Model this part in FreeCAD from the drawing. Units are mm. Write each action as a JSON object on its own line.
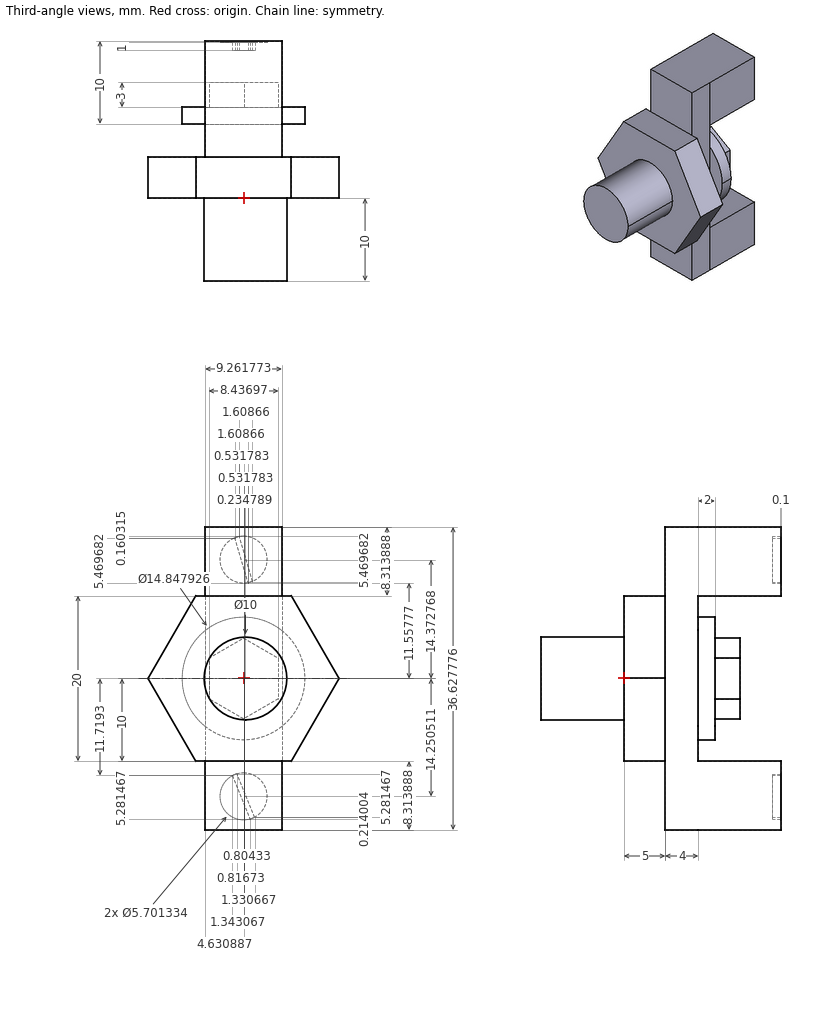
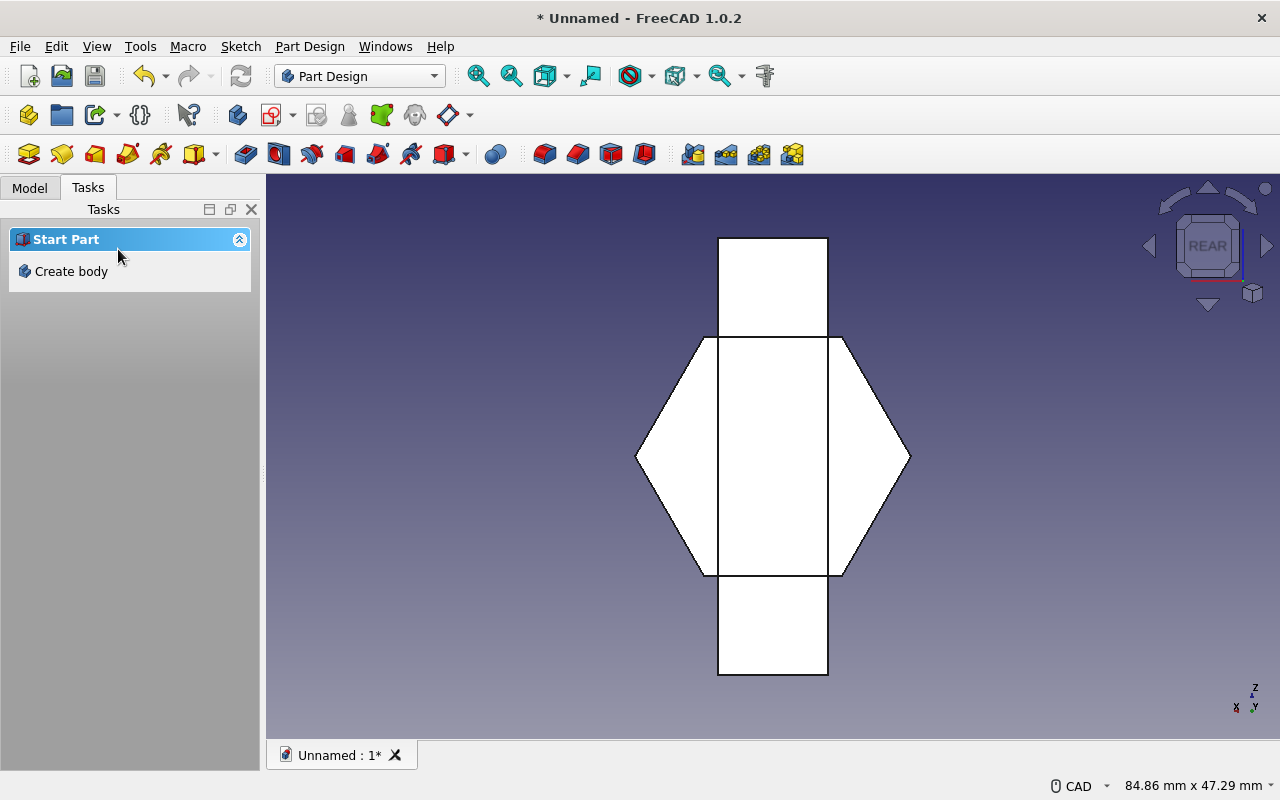
{"action": "left_click", "coordinate": [773, 455]}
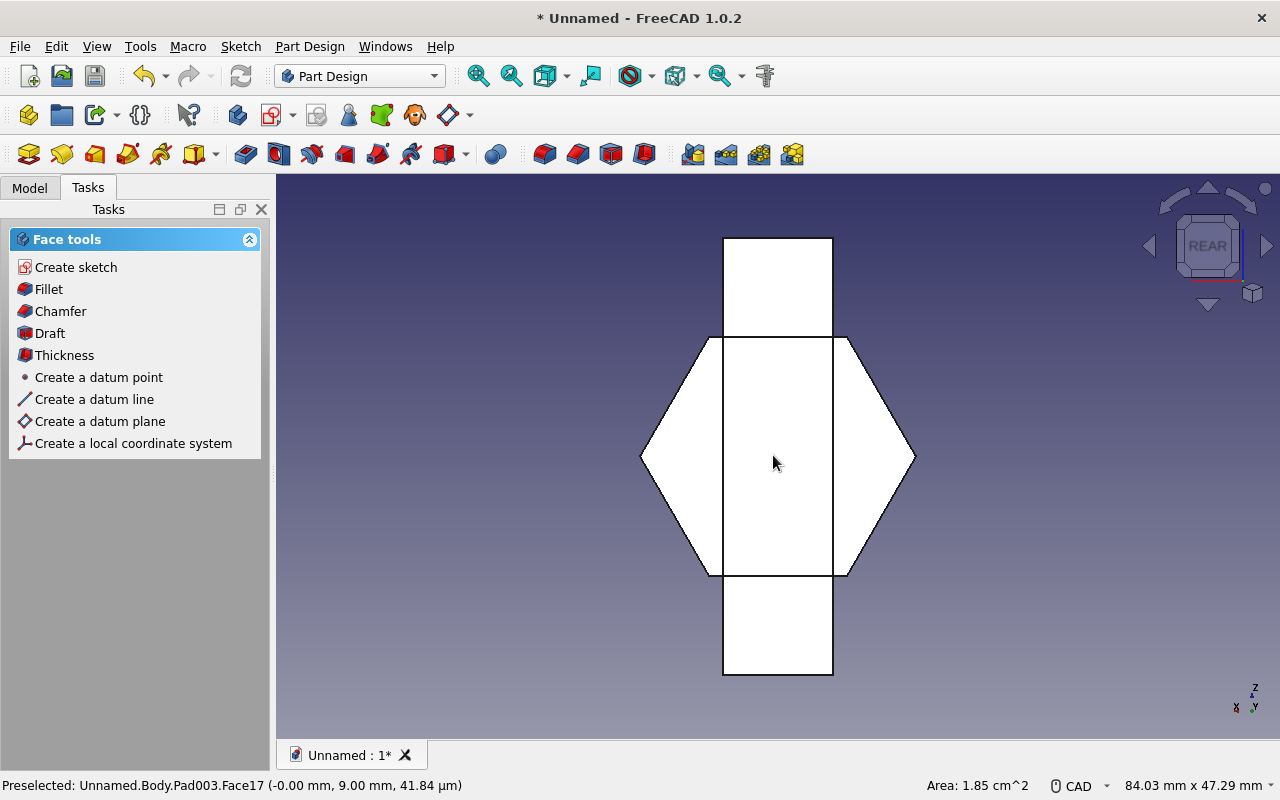
{"action": "left_click", "coordinate": [270, 116]}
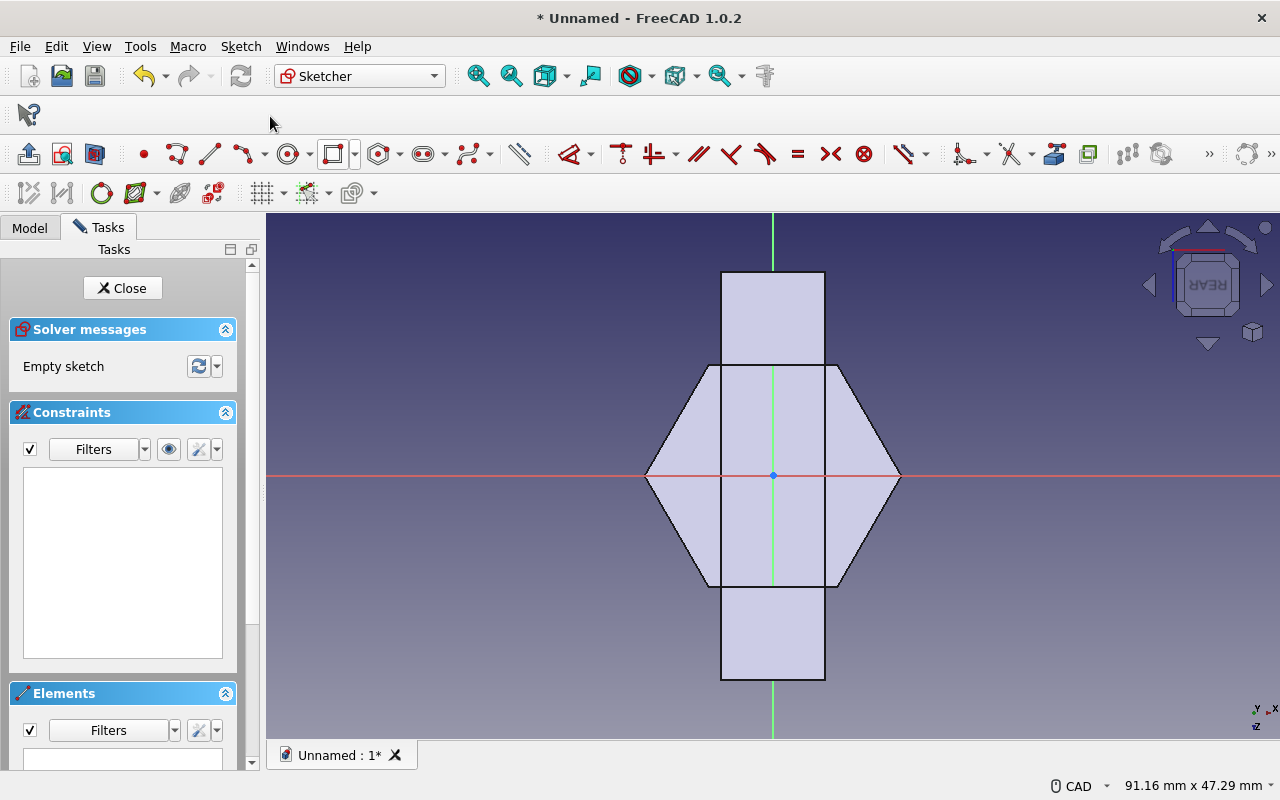
{"action": "scroll", "coordinate": [856, 476], "scroll_direction": "up", "scroll_amount": 3}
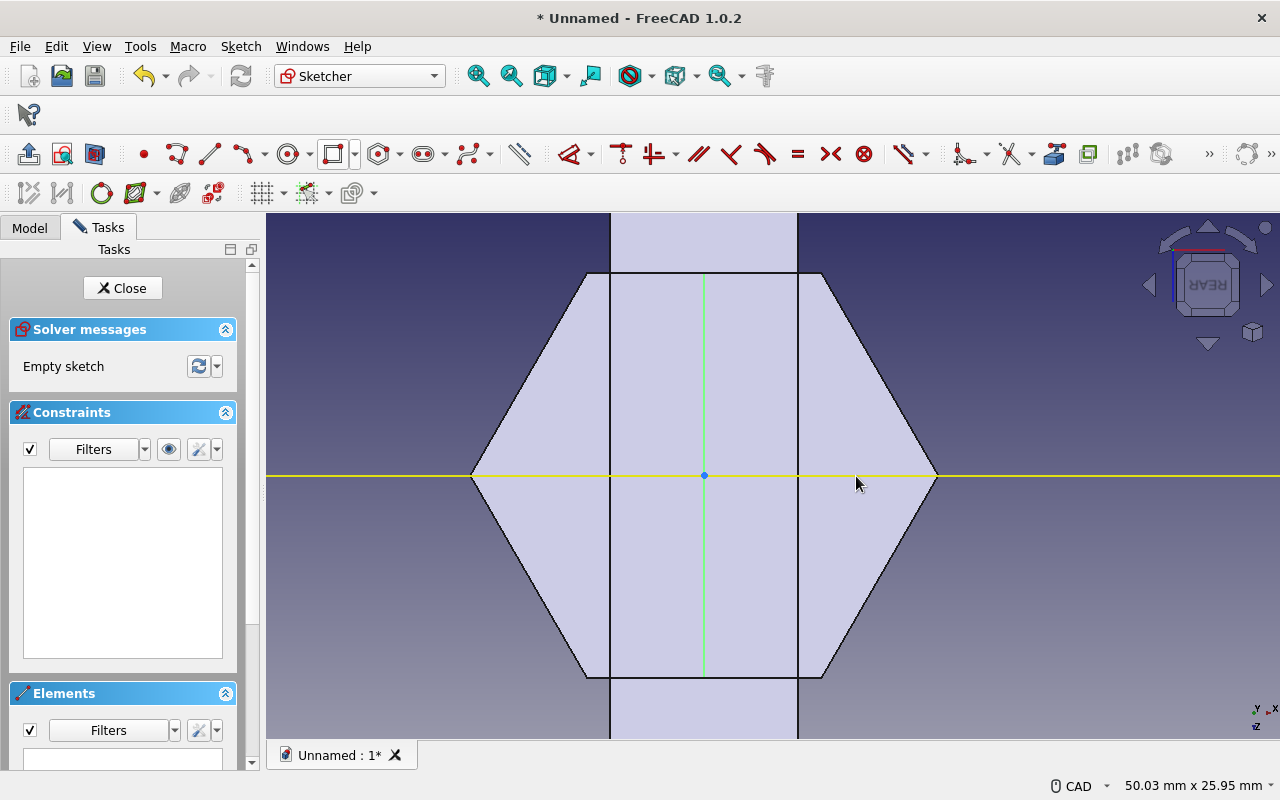
{"action": "left_click", "coordinate": [288, 154]}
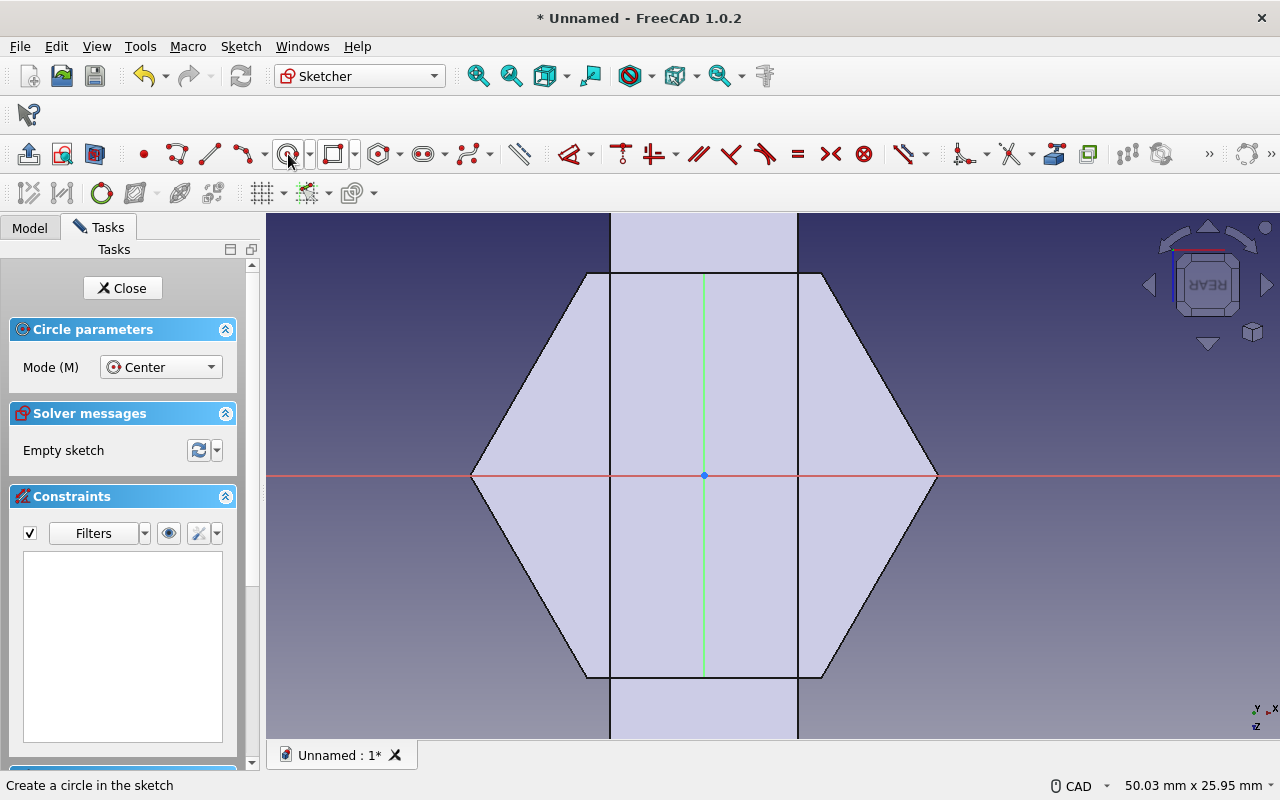
{"action": "left_click", "coordinate": [704, 476]}
{"action": "mouse_move", "coordinate": [811, 369]}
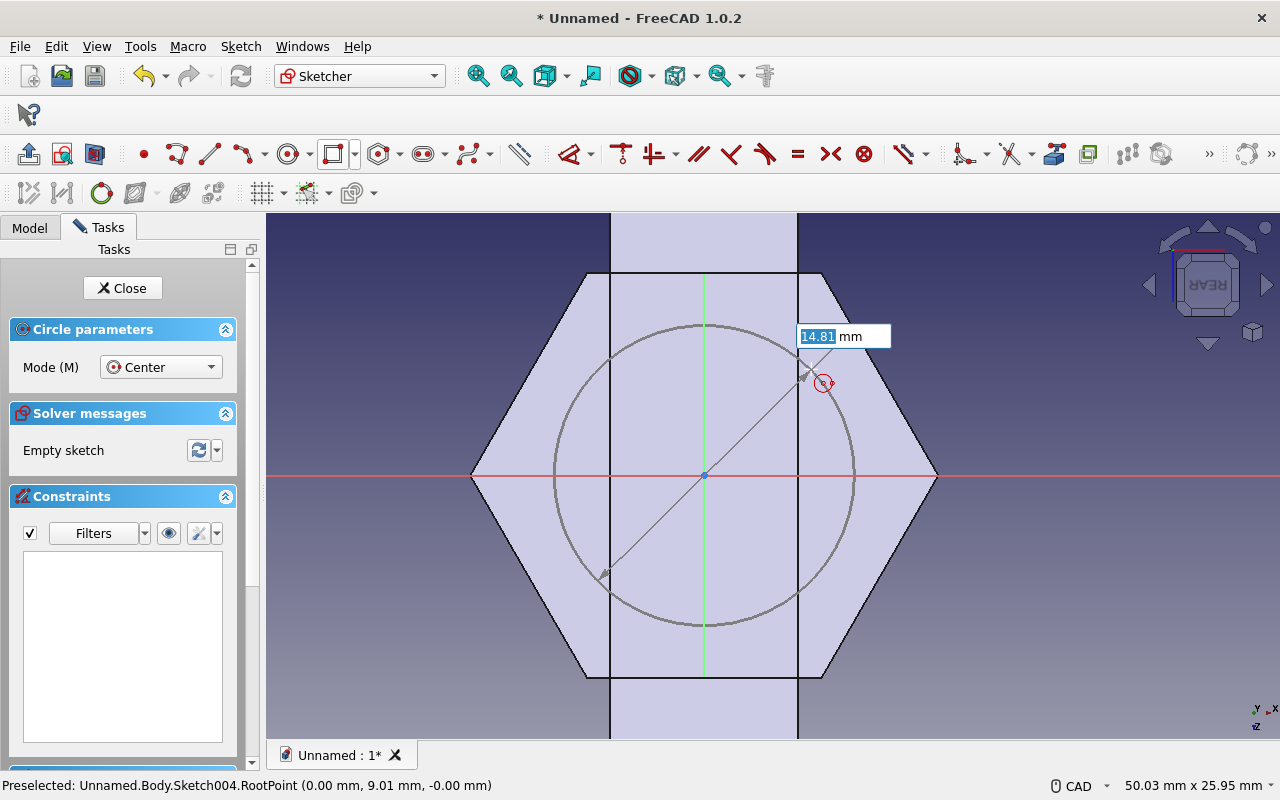
{"action": "type", "text": "14.847926"}
{"action": "key", "text": "Return"}
{"action": "key", "text": "Escape"}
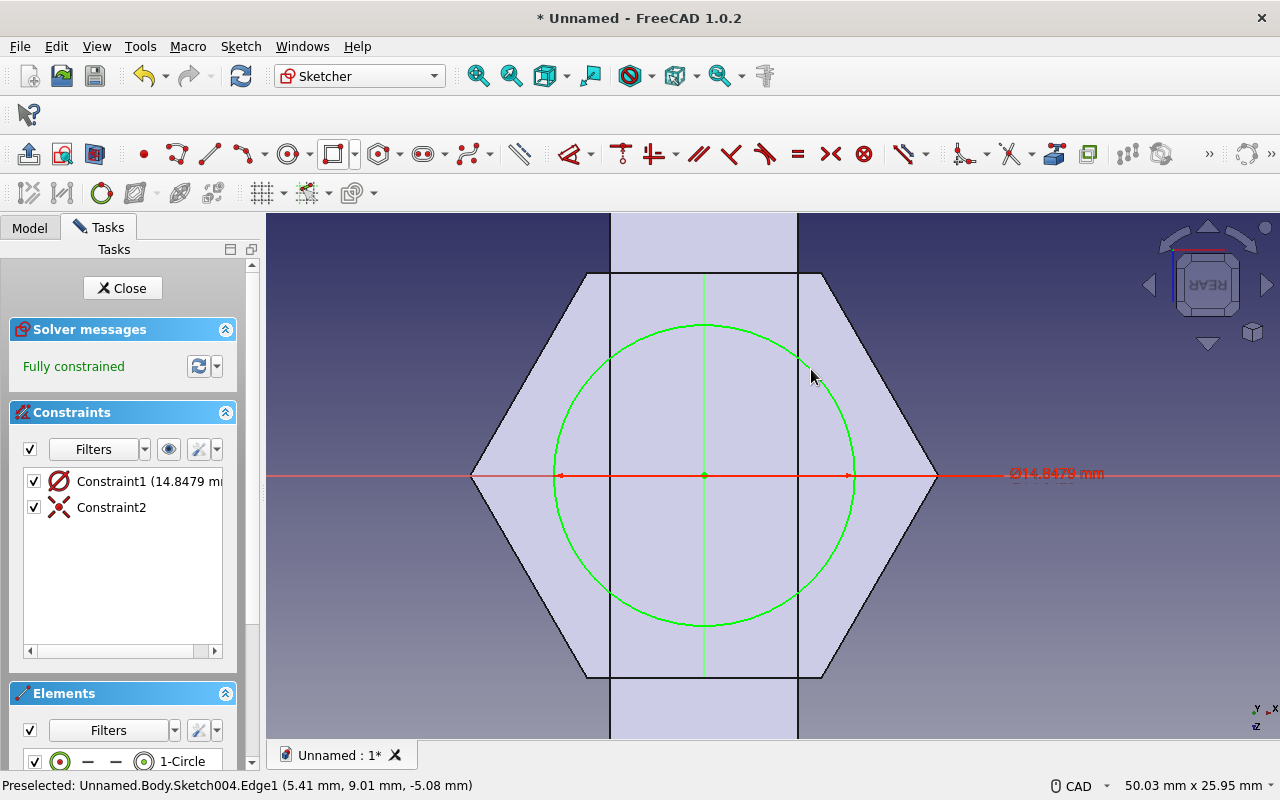
{"action": "left_click", "coordinate": [123, 288]}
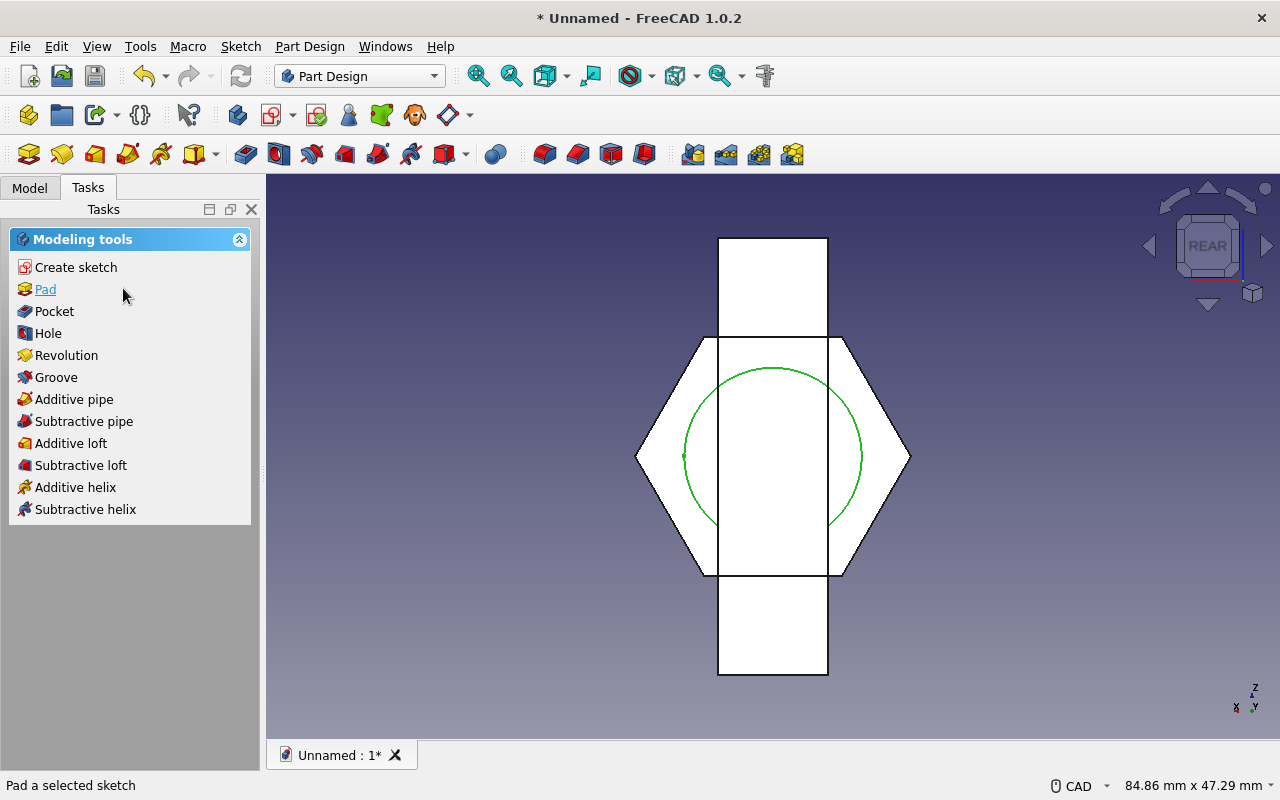
{"action": "left_click", "coordinate": [29, 154]}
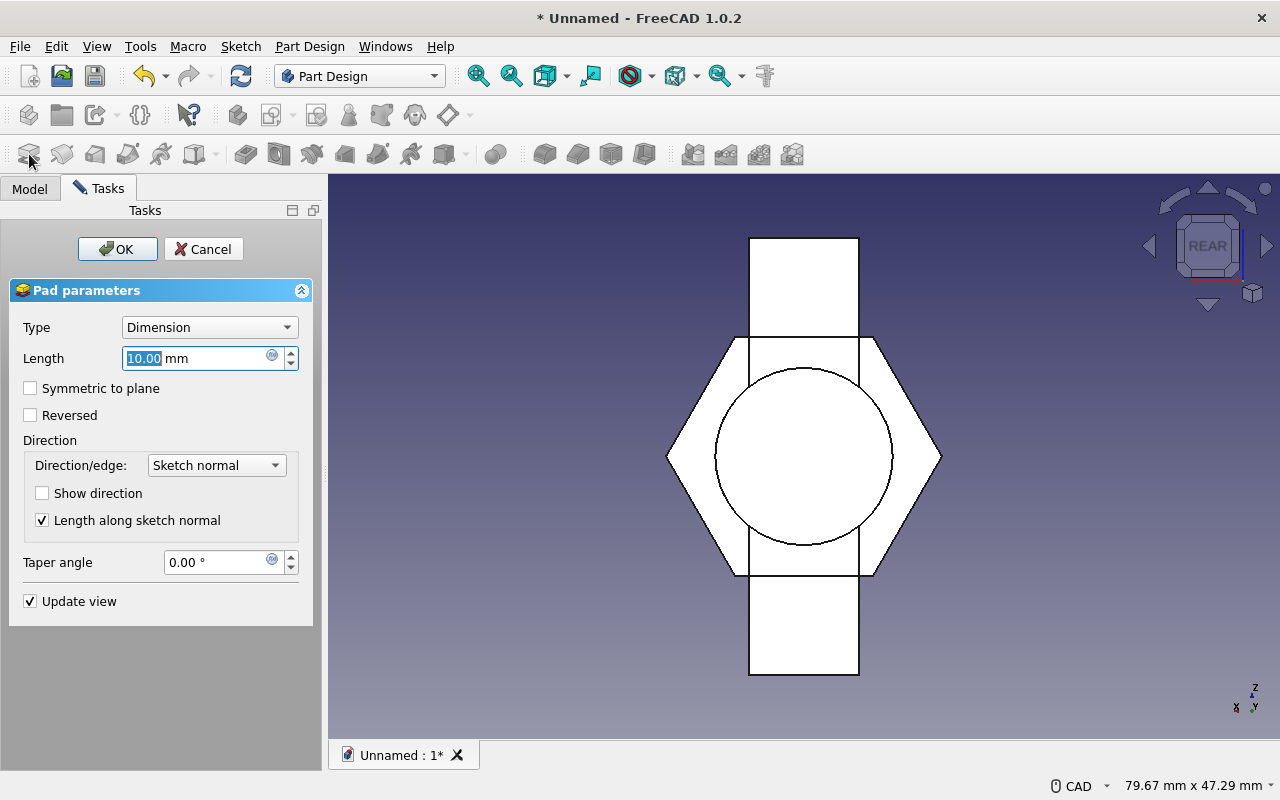
{"action": "type", "text": "2"}
{"action": "key", "text": "Tab"}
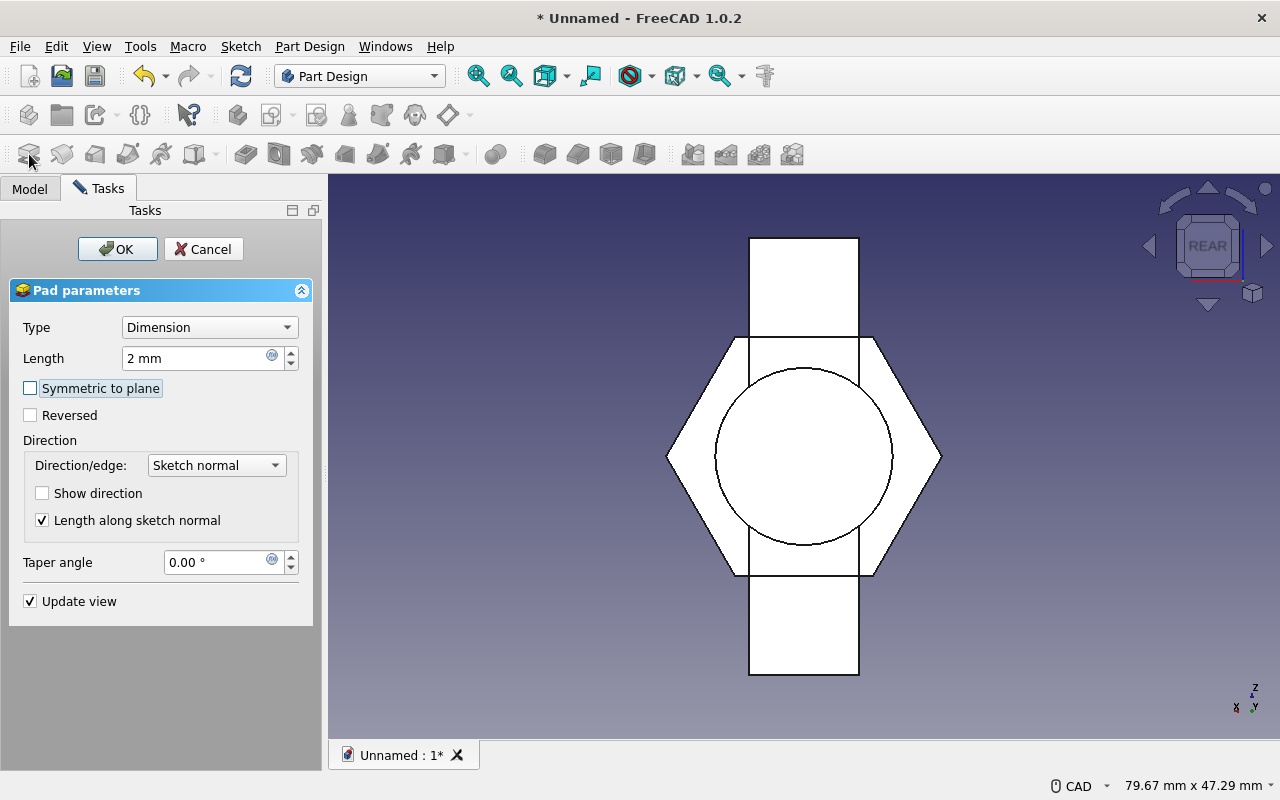
{"action": "left_click", "coordinate": [118, 249]}